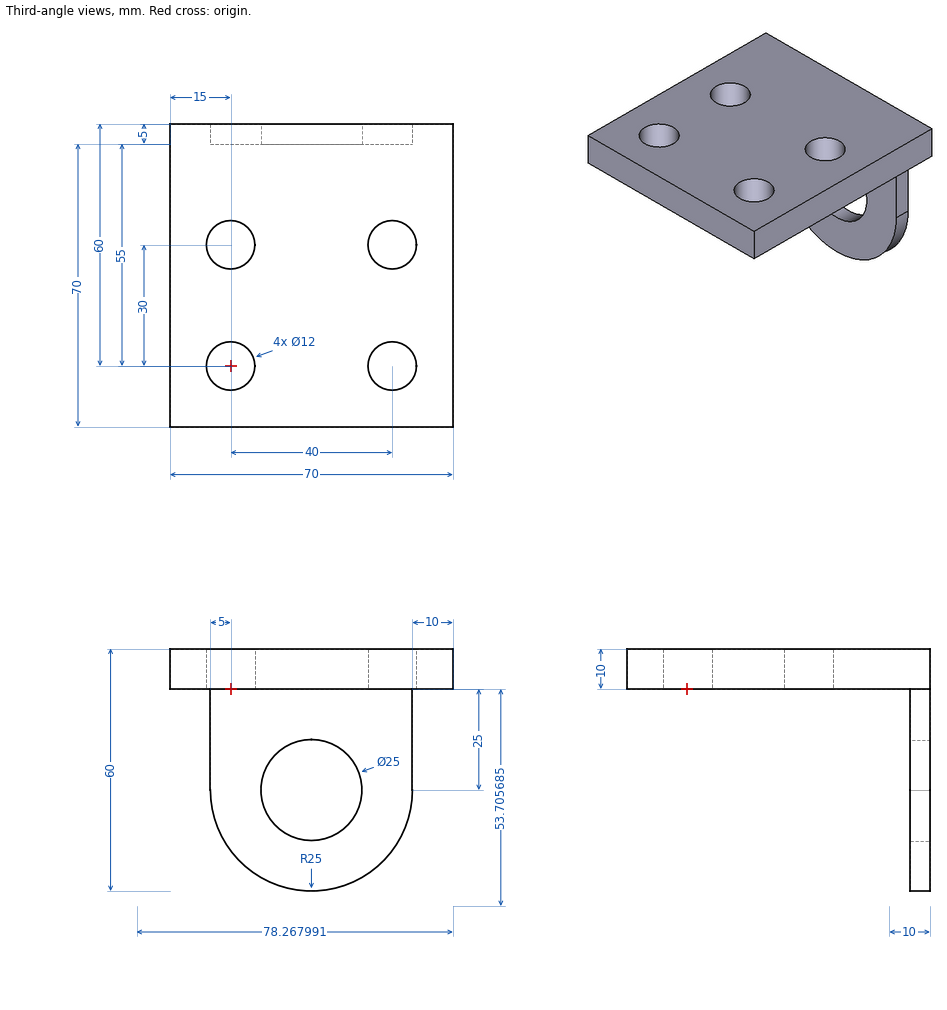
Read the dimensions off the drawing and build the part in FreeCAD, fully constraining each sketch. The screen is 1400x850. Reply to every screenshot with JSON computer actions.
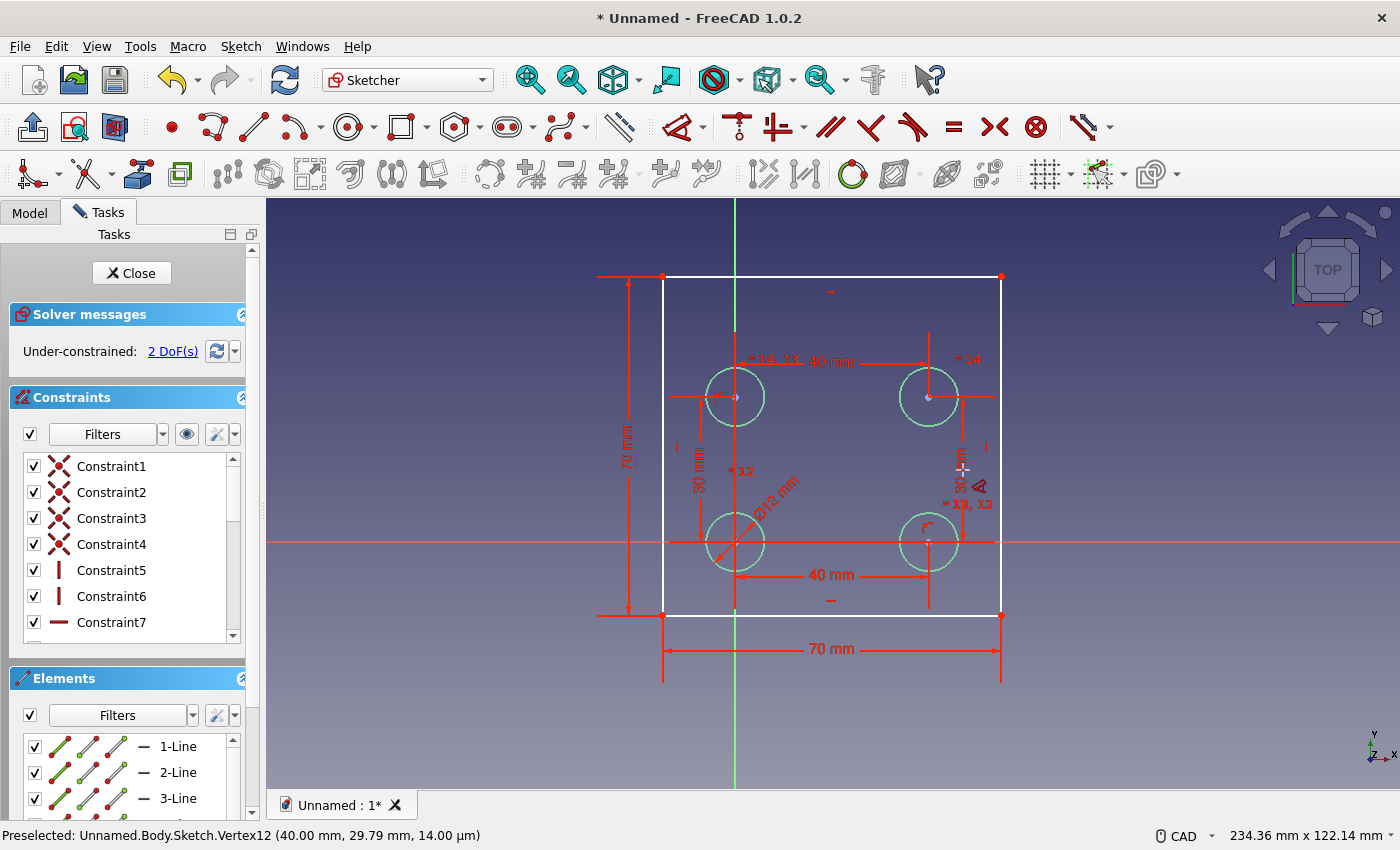
{"action": "left_click", "coordinate": [663, 277]}
{"action": "left_click", "coordinate": [699, 243]}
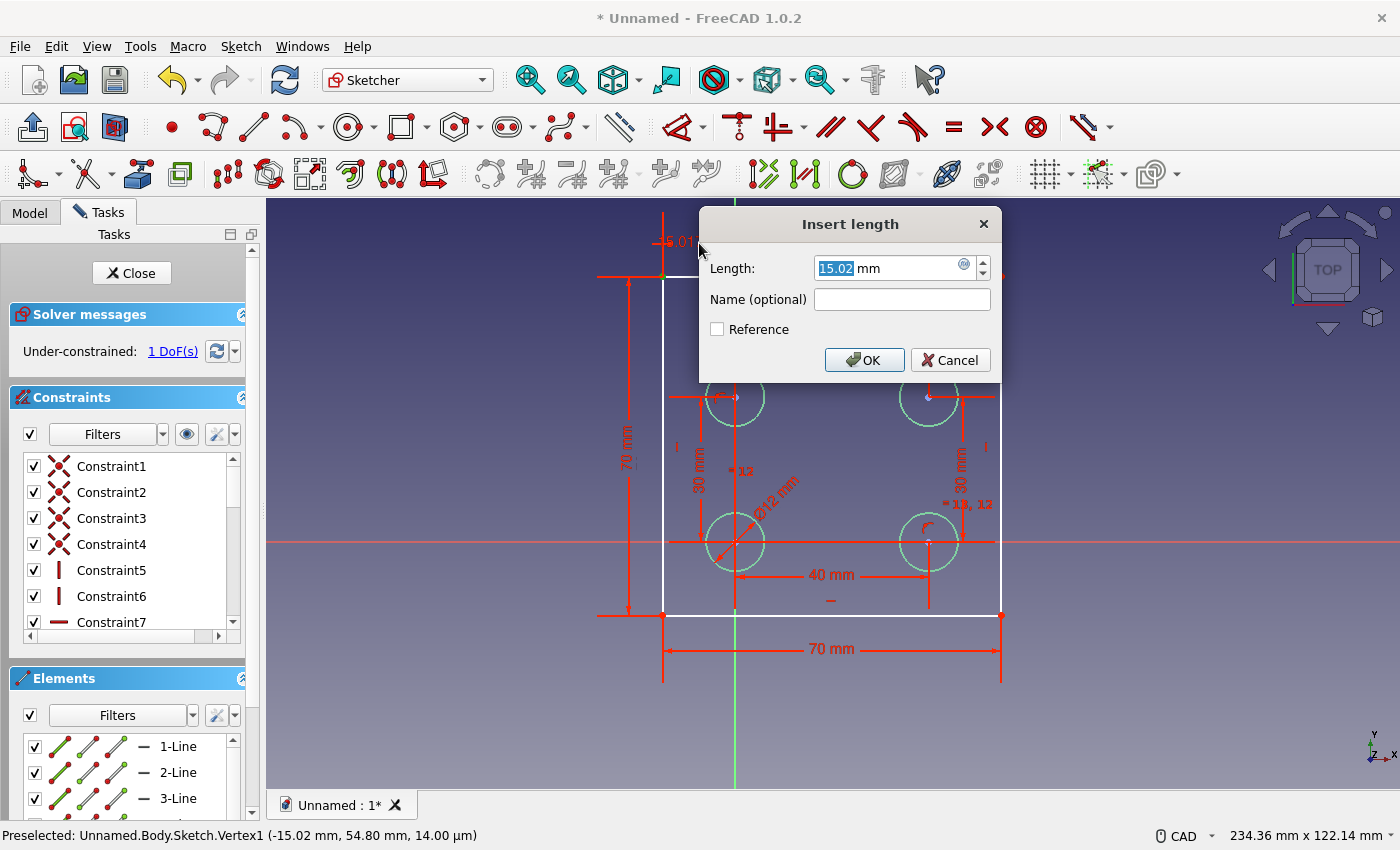
{"action": "type", "text": "15"}
{"action": "key", "text": "Return"}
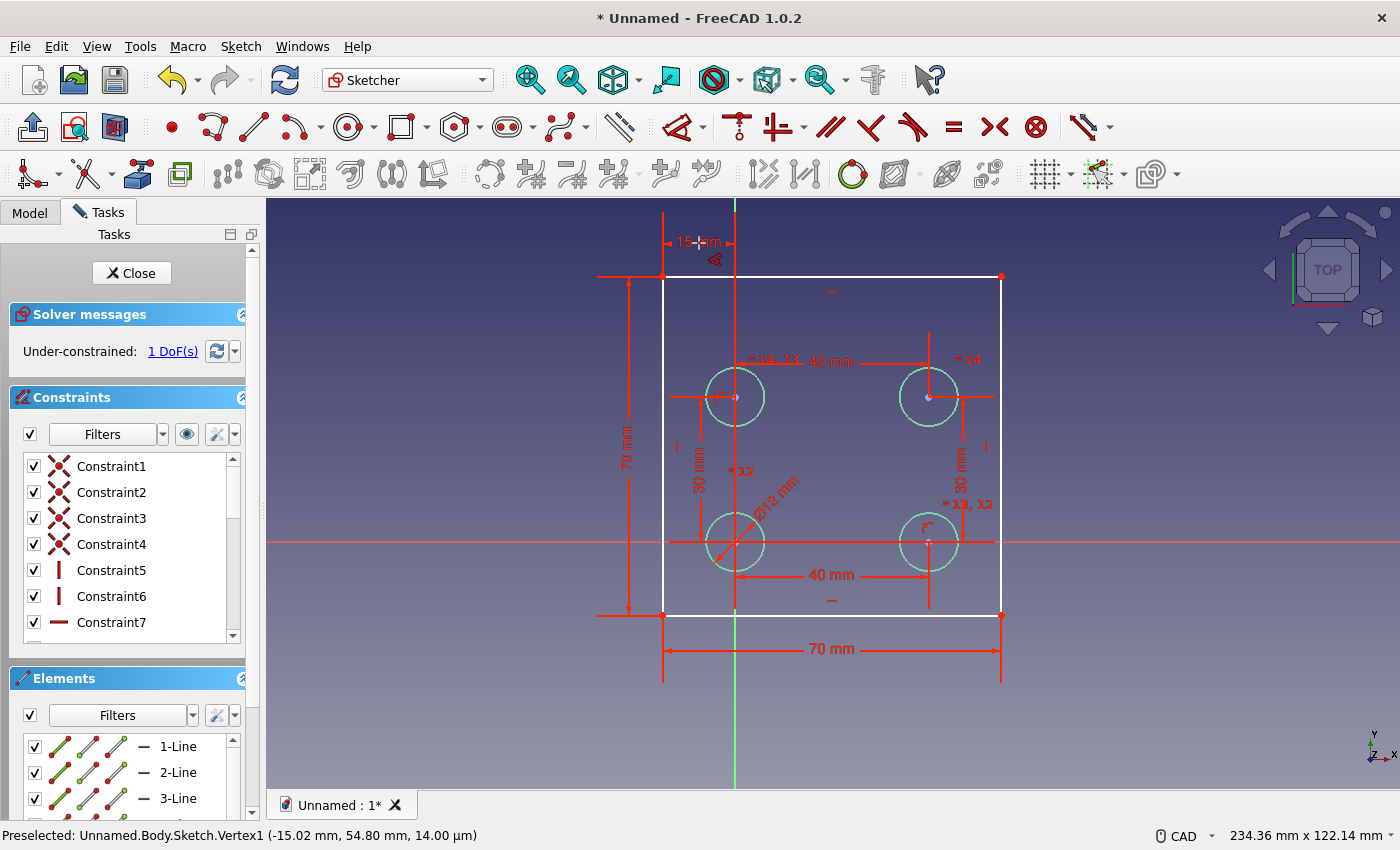
{"action": "left_click", "coordinate": [663, 277]}
{"action": "left_click", "coordinate": [629, 410]}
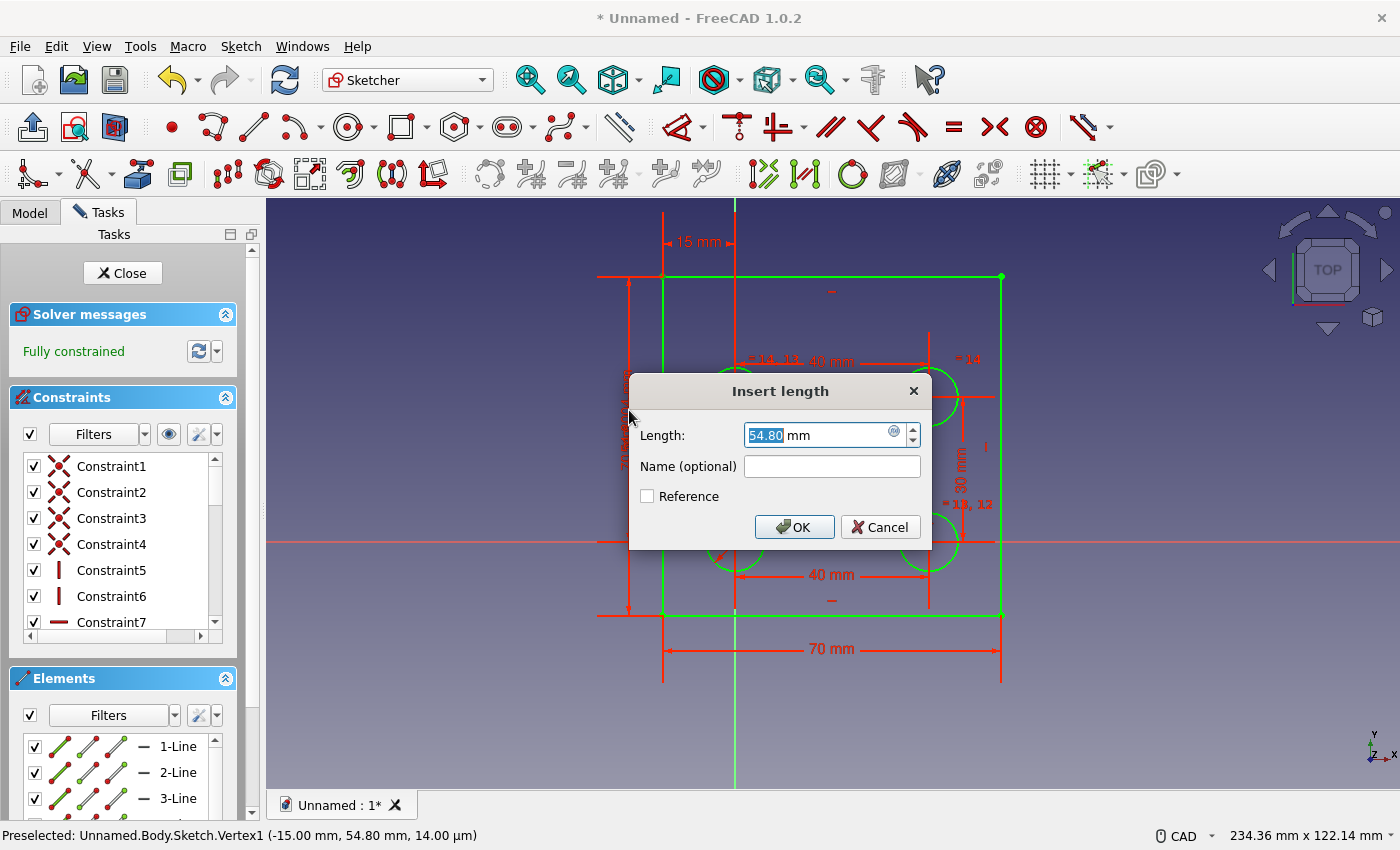
{"action": "type", "text": "55"}
{"action": "key", "text": "Return"}
{"action": "key", "text": "Escape"}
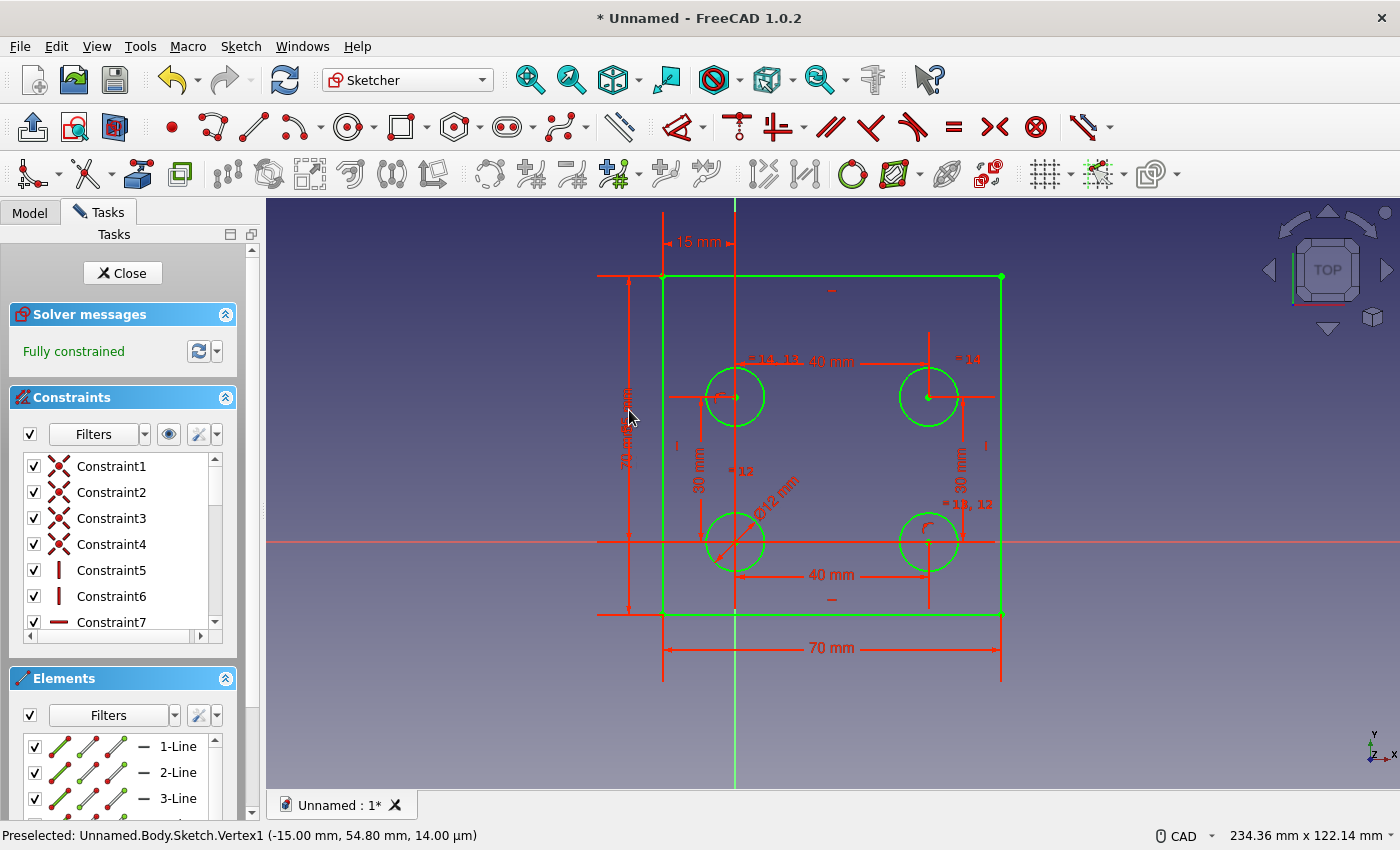
{"action": "left_click", "coordinate": [123, 273]}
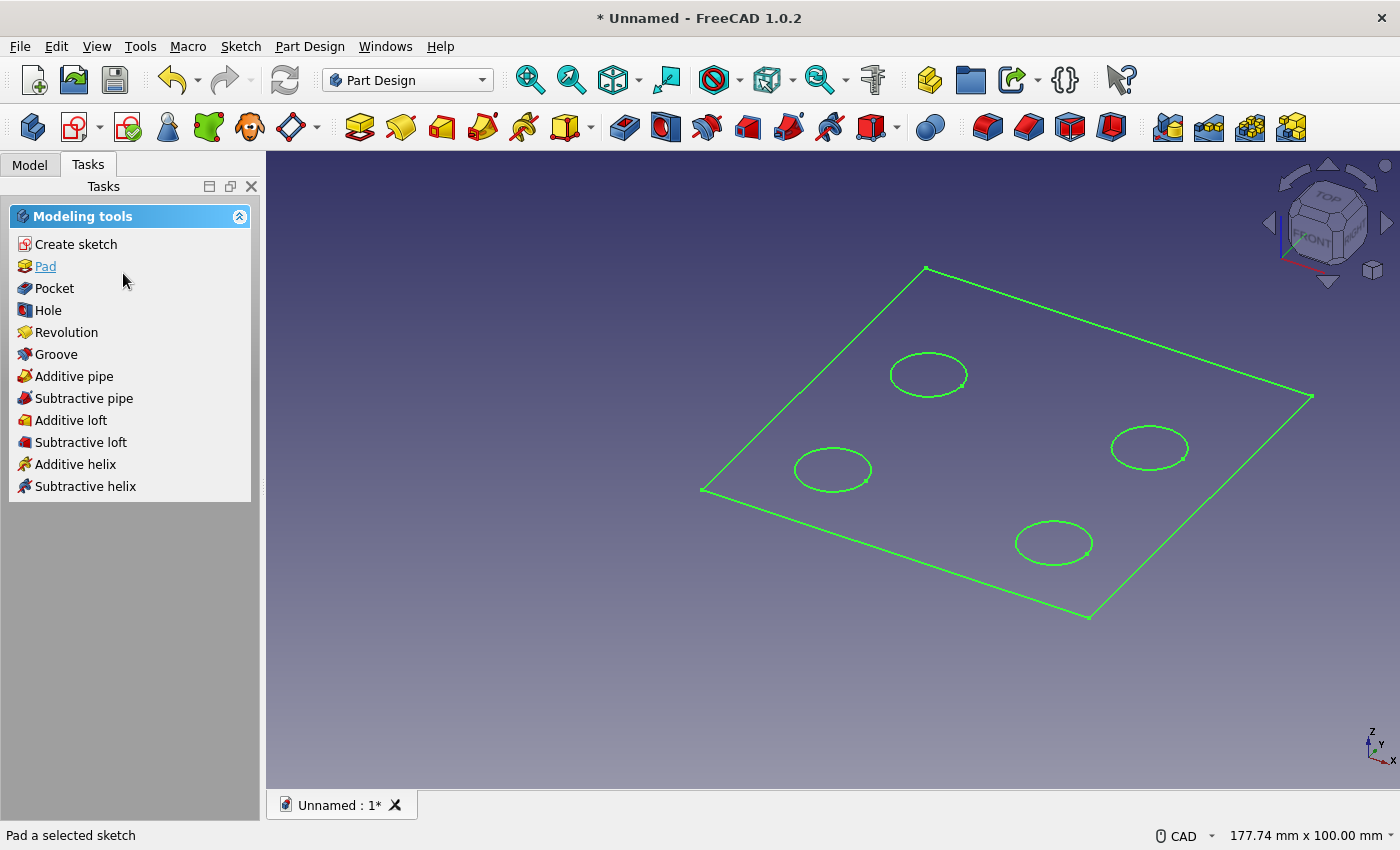
{"action": "left_click", "coordinate": [360, 128]}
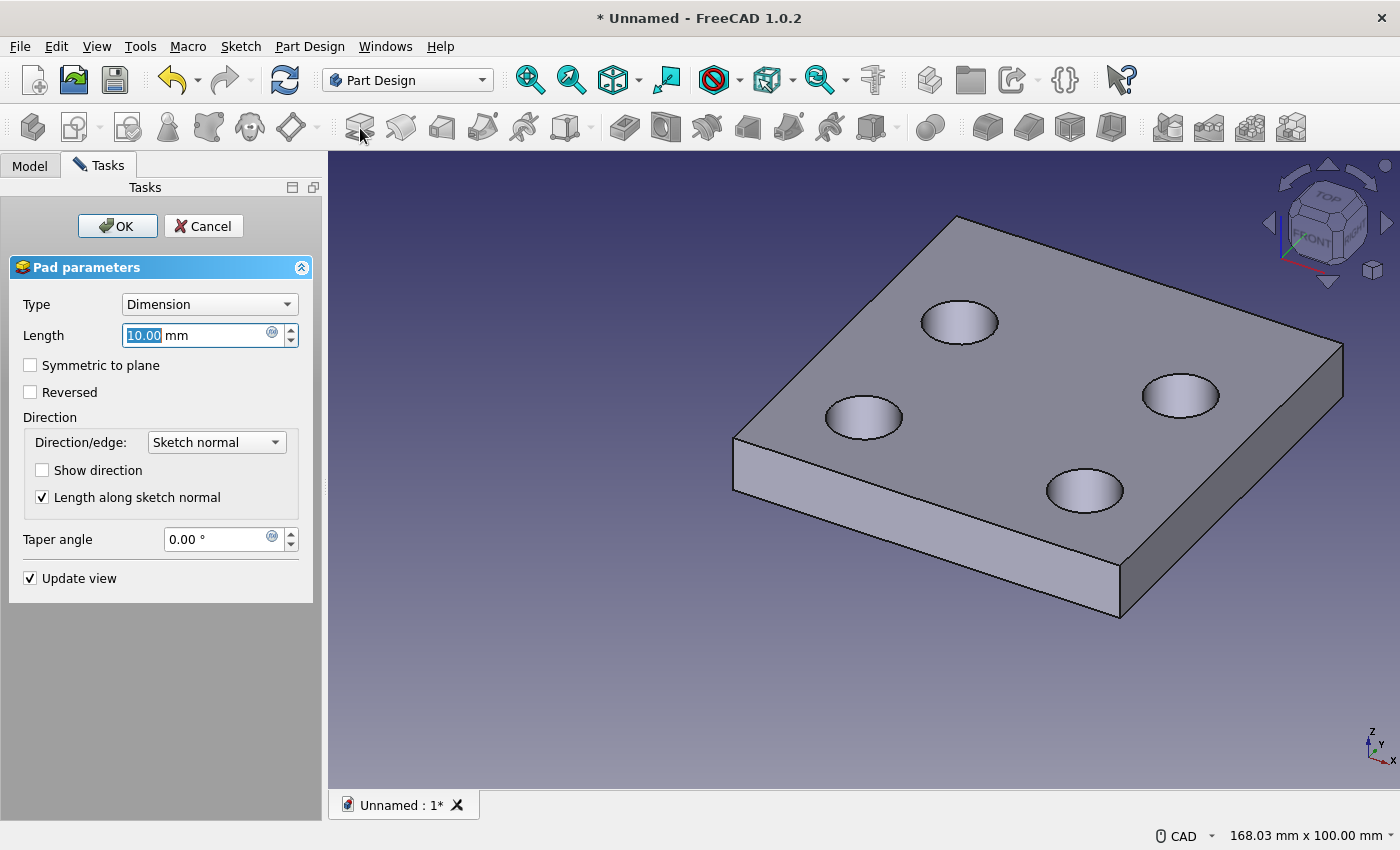
{"action": "type", "text": "10"}
{"action": "key", "text": "Tab"}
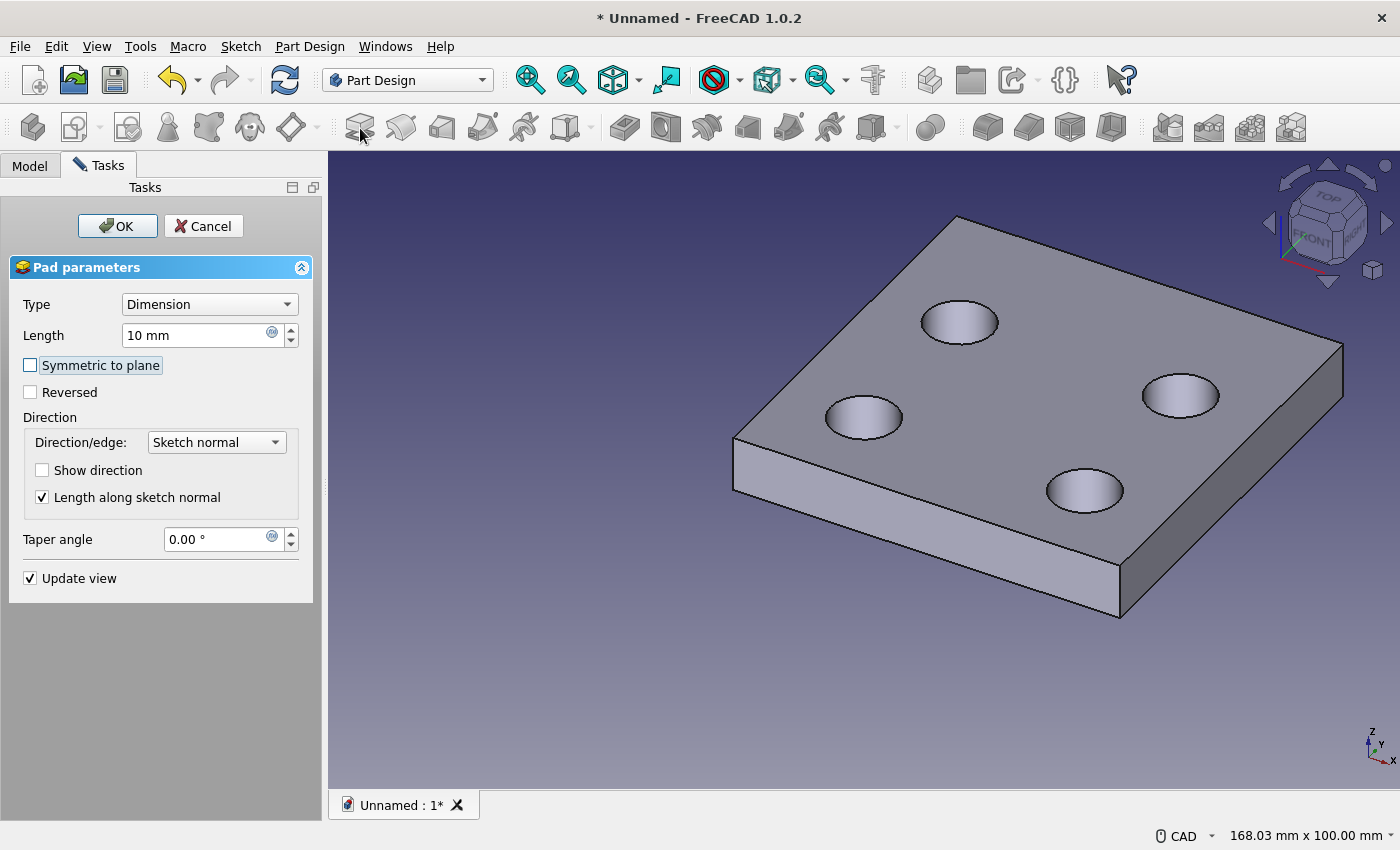
{"action": "left_click", "coordinate": [118, 226]}